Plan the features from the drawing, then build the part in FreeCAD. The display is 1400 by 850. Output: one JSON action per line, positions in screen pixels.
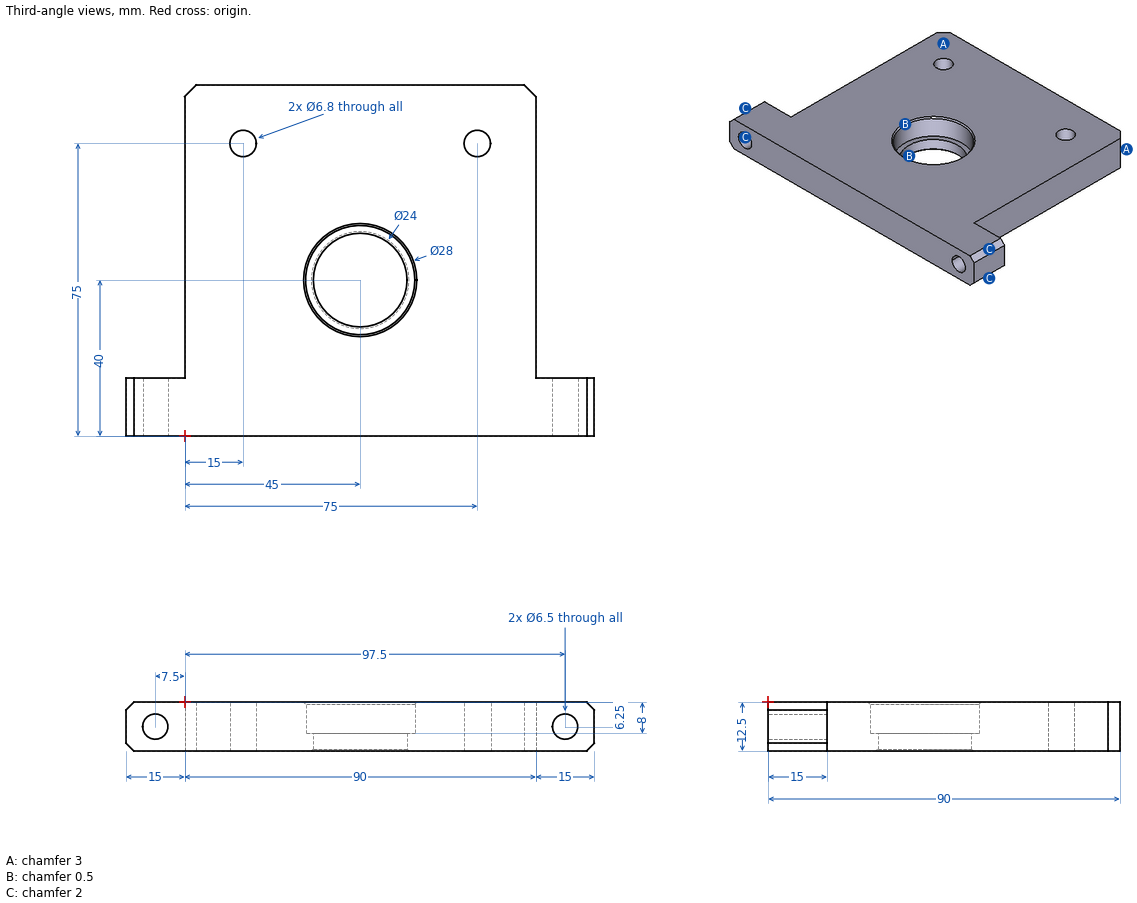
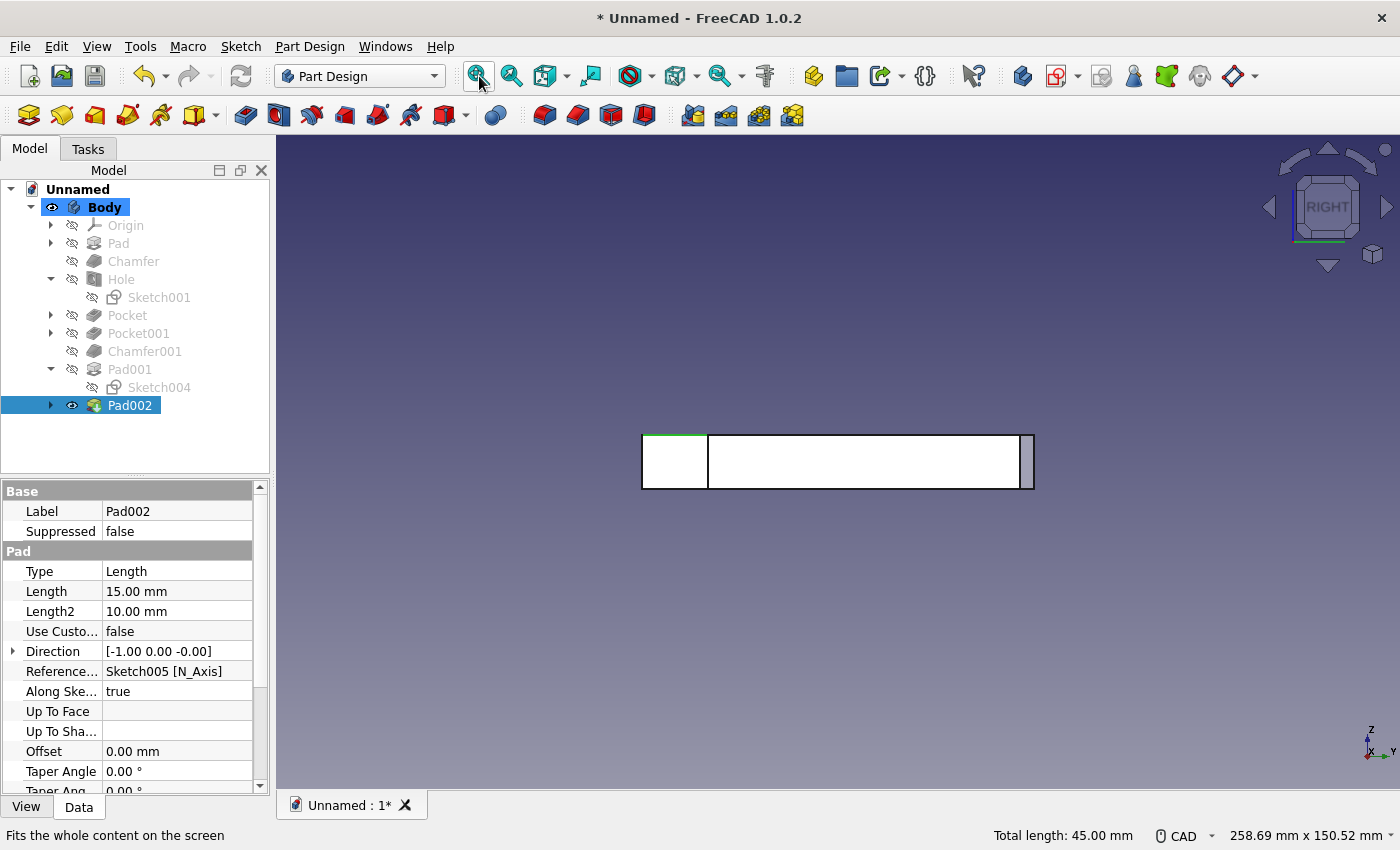
{"action": "left_click", "coordinate": [675, 488], "text": "ctrl"}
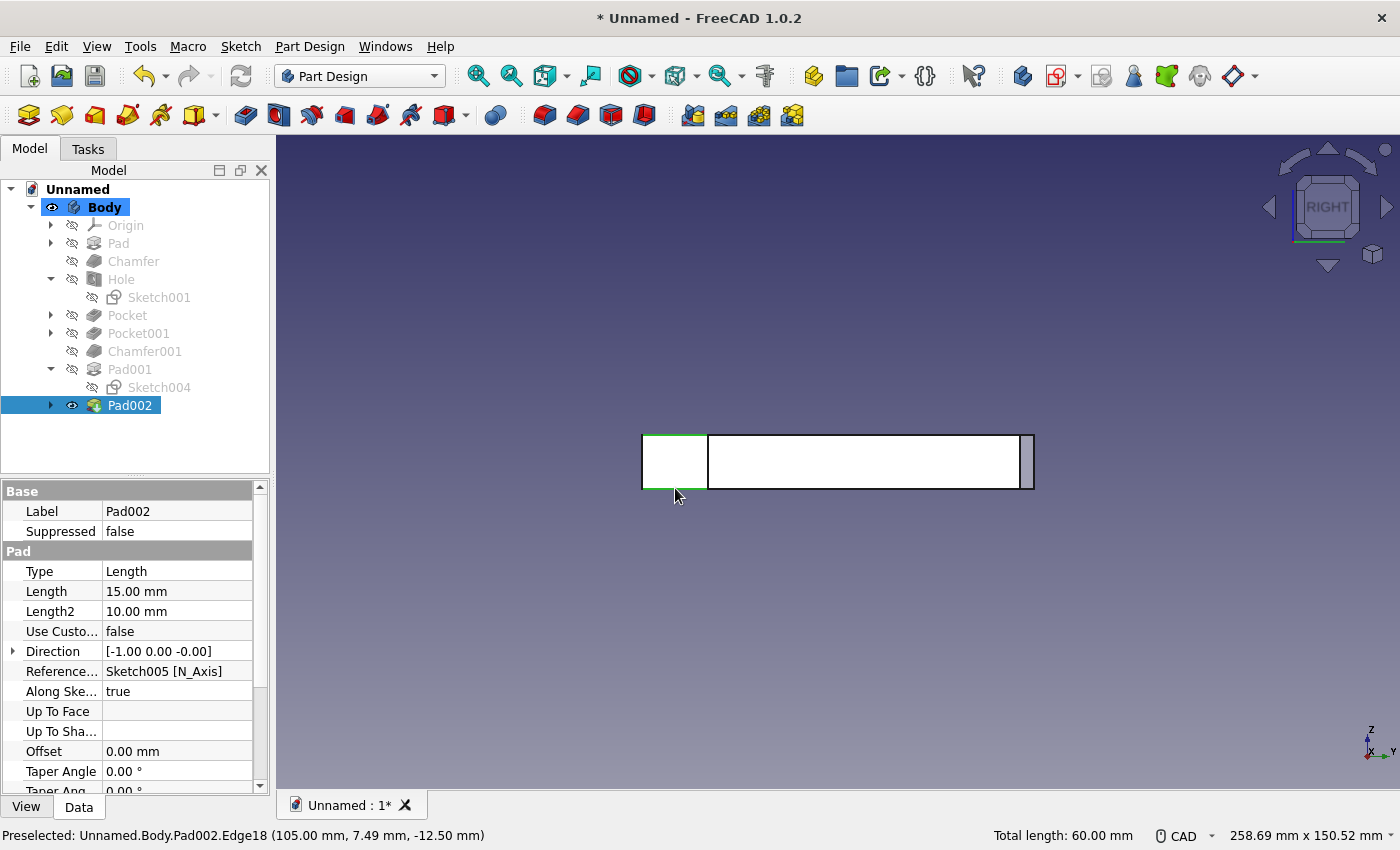
{"action": "left_click", "coordinate": [578, 116]}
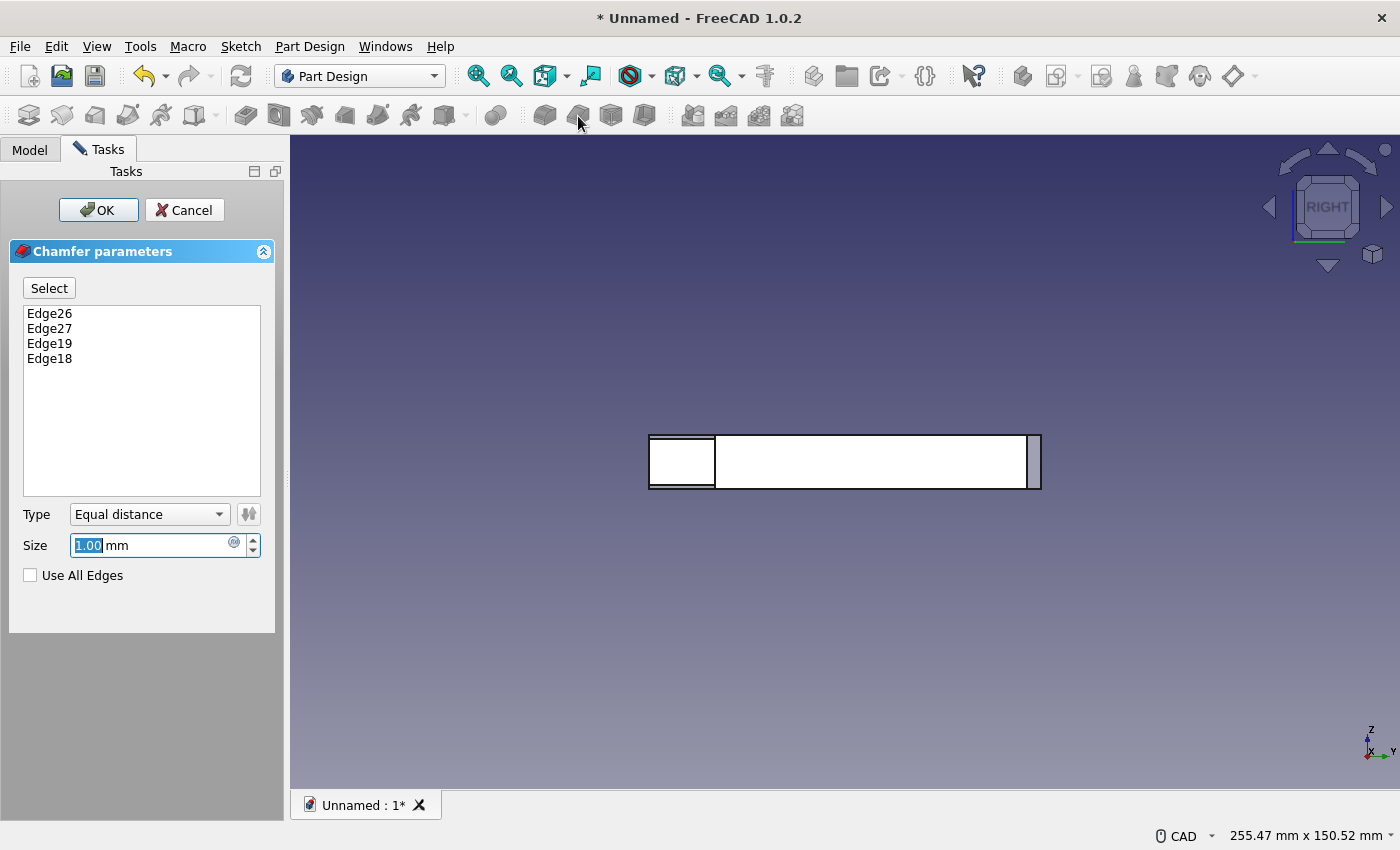
{"action": "type", "text": "2"}
{"action": "key", "text": "Tab"}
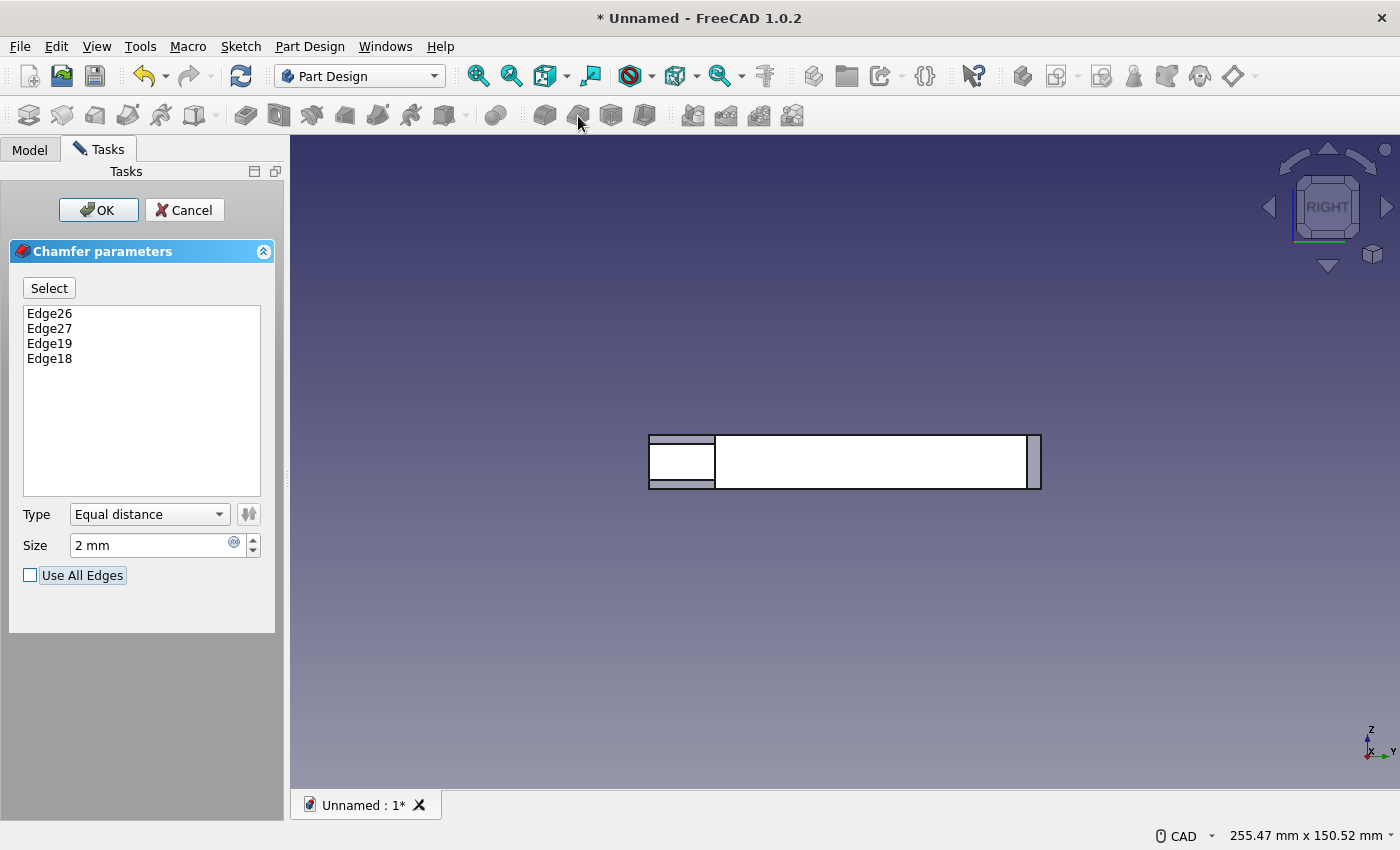
{"action": "left_click", "coordinate": [99, 210]}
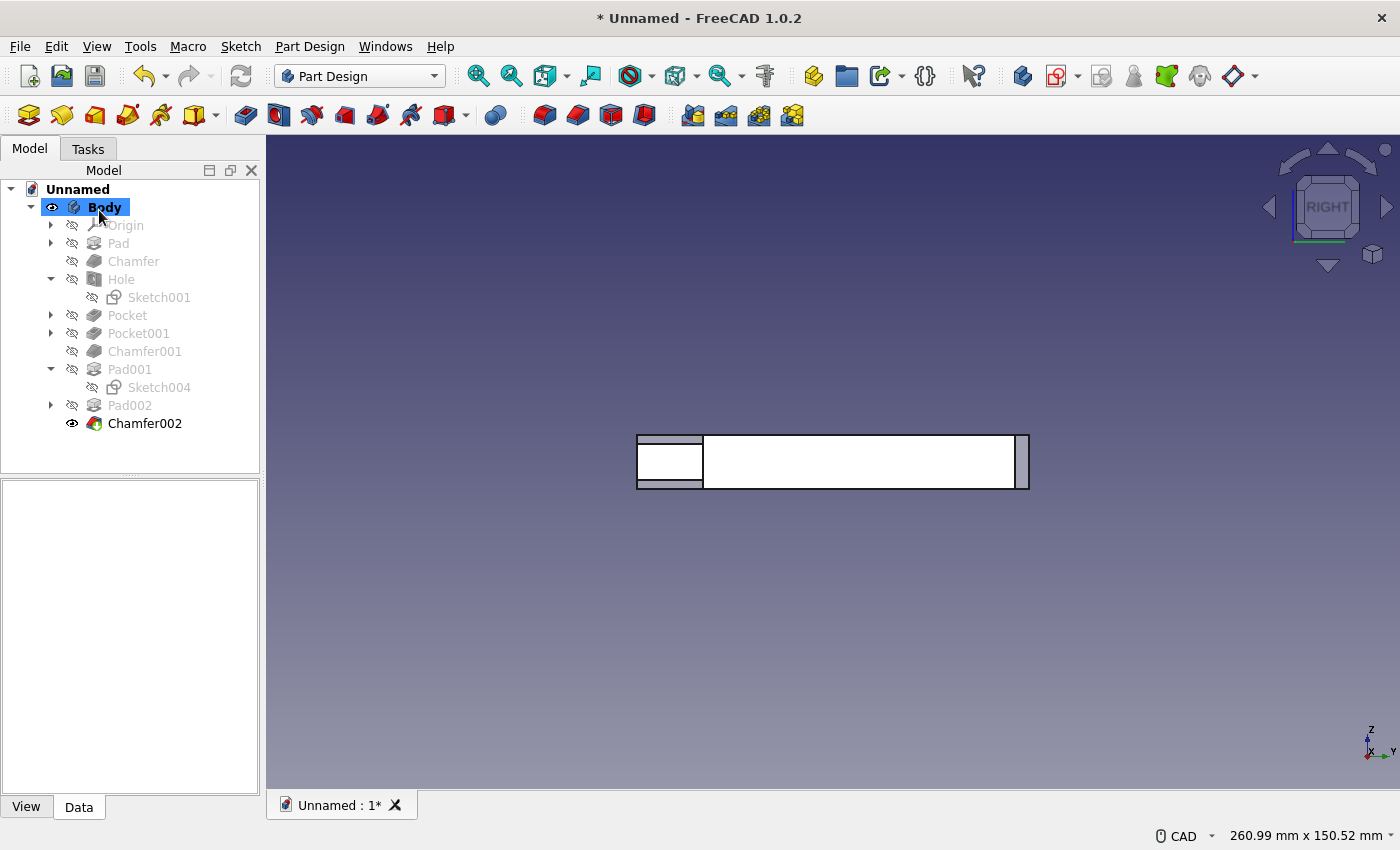
{"action": "left_click", "coordinate": [479, 76]}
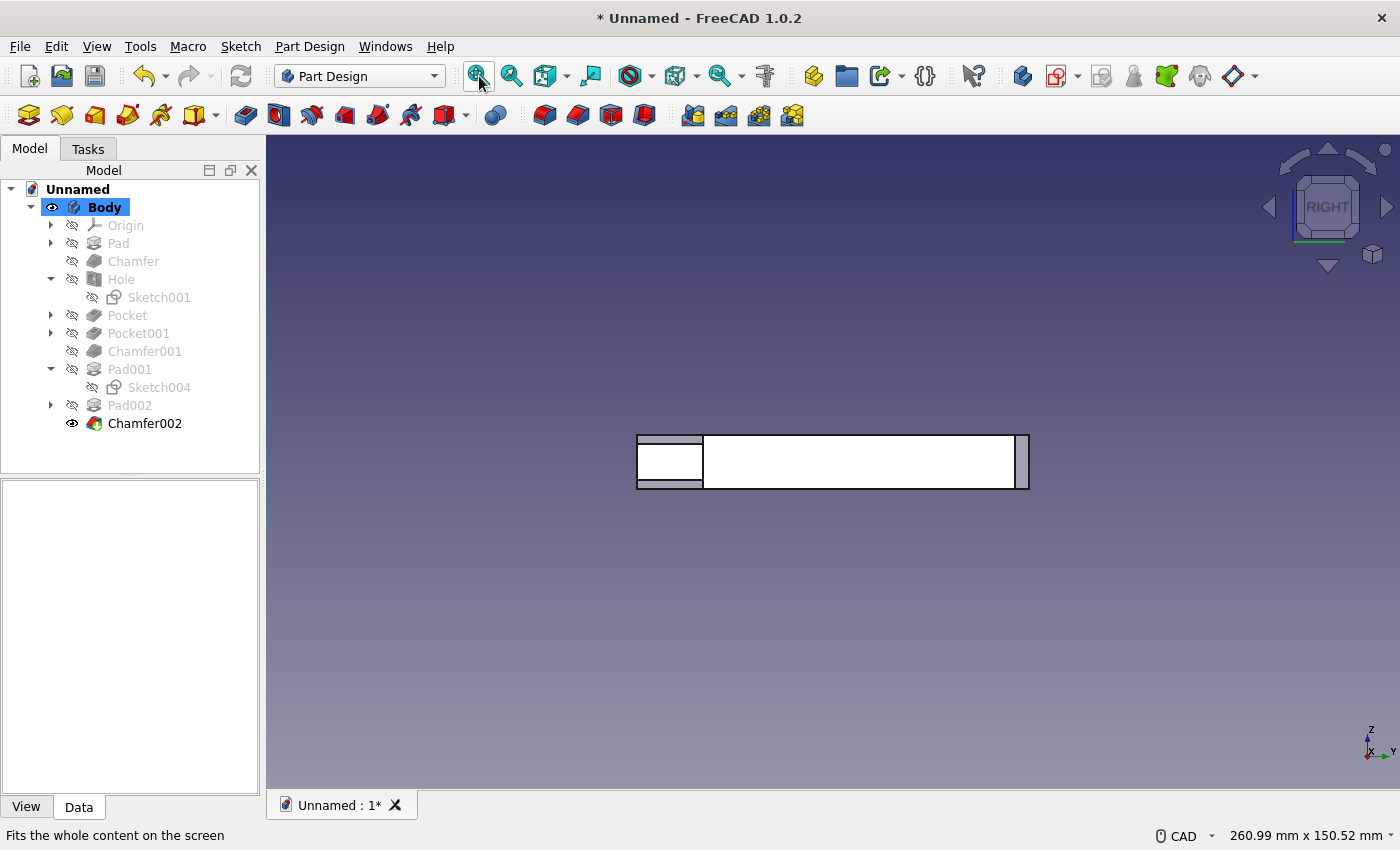
{"action": "key", "text": "4"}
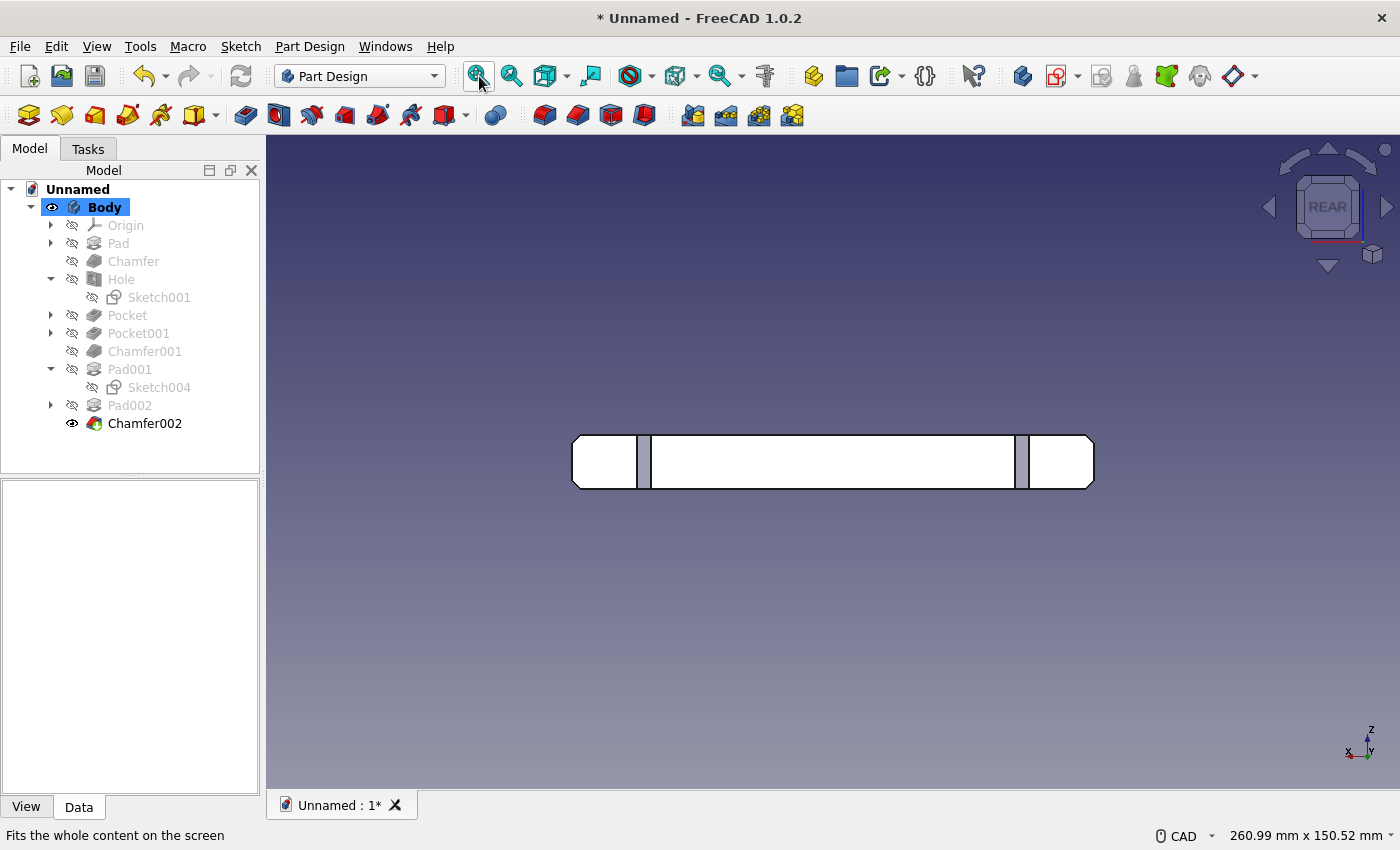
{"action": "left_click", "coordinate": [1061, 461]}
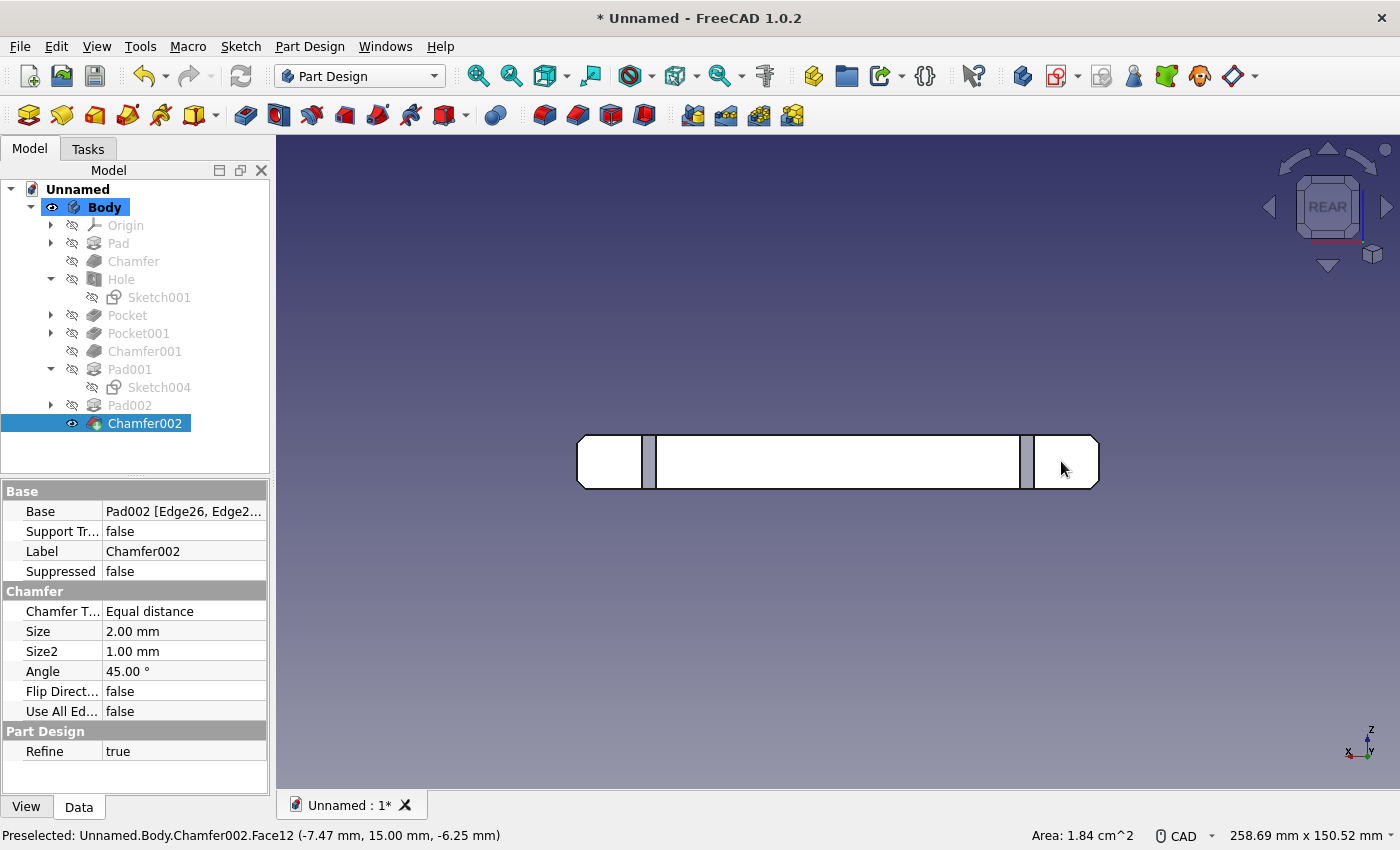
{"action": "left_click", "coordinate": [1056, 76]}